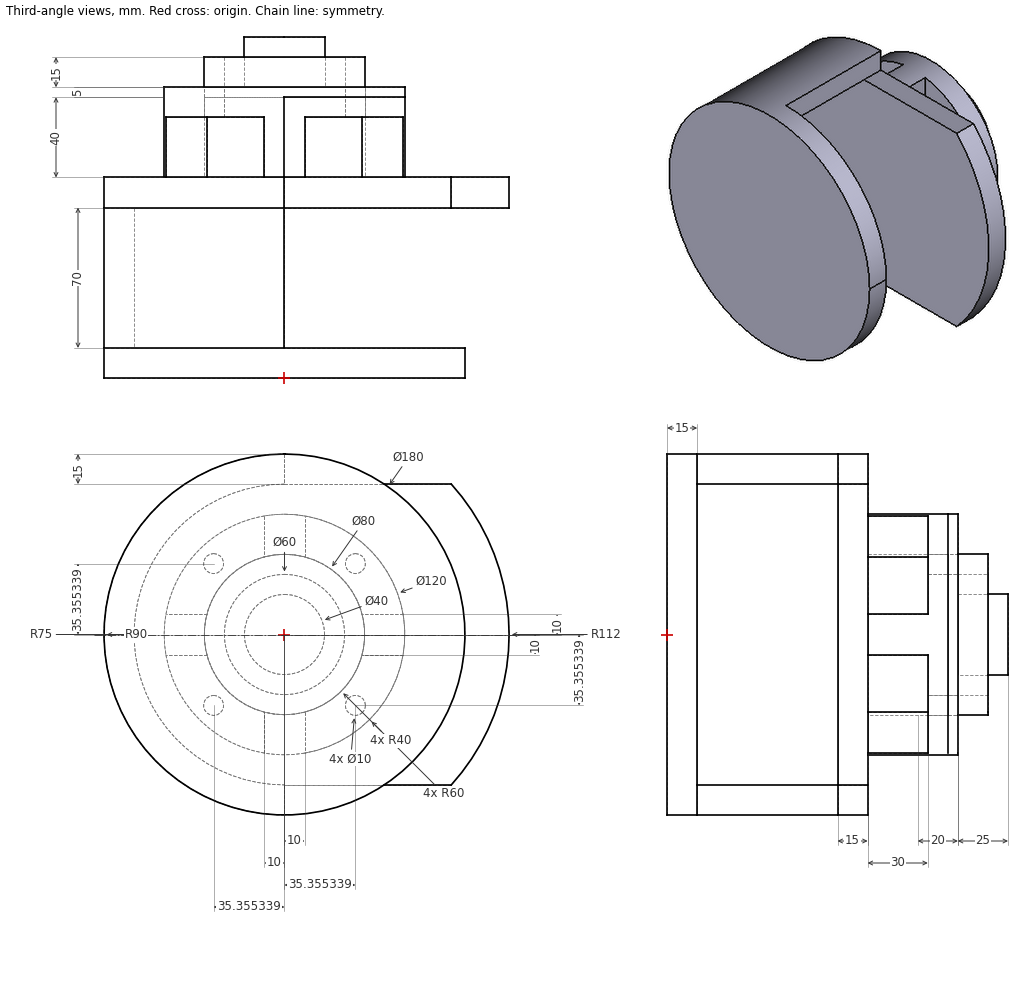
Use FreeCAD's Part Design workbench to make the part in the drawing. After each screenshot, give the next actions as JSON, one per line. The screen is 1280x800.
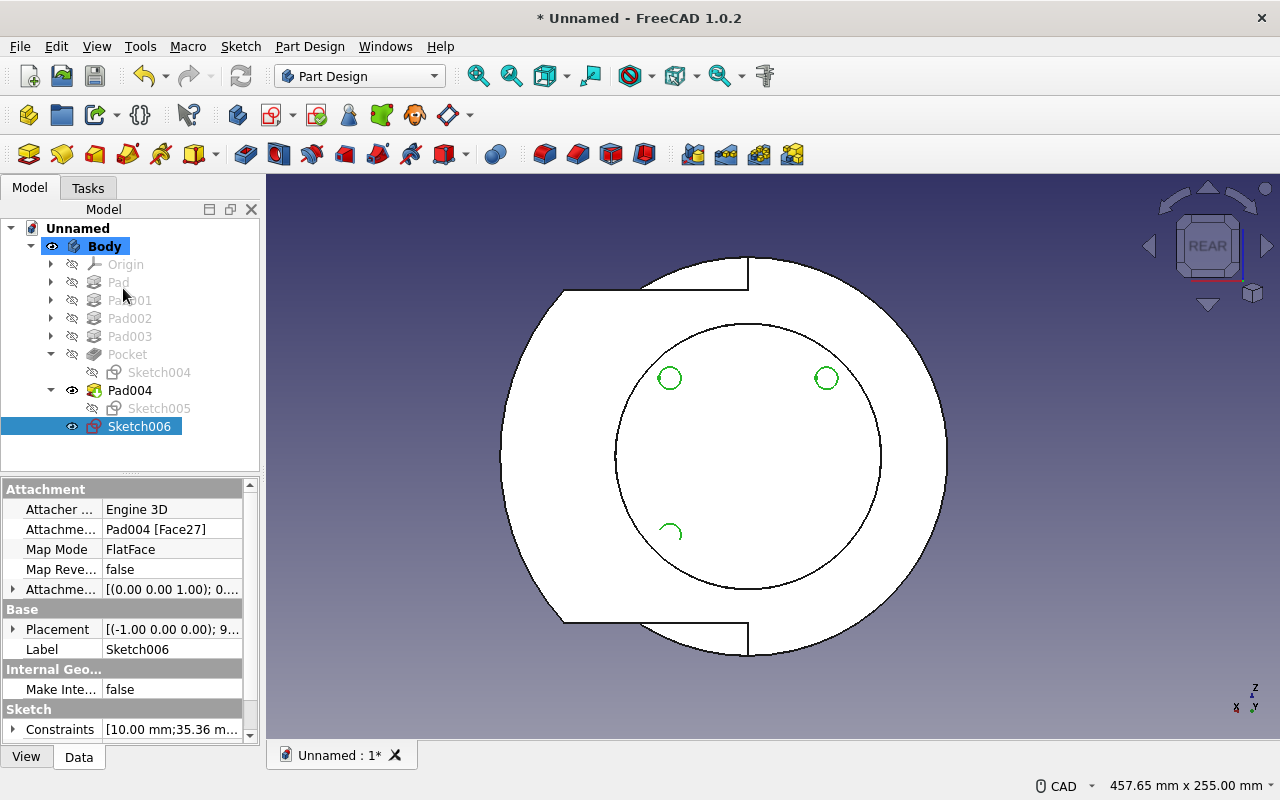
{"action": "left_click", "coordinate": [246, 154]}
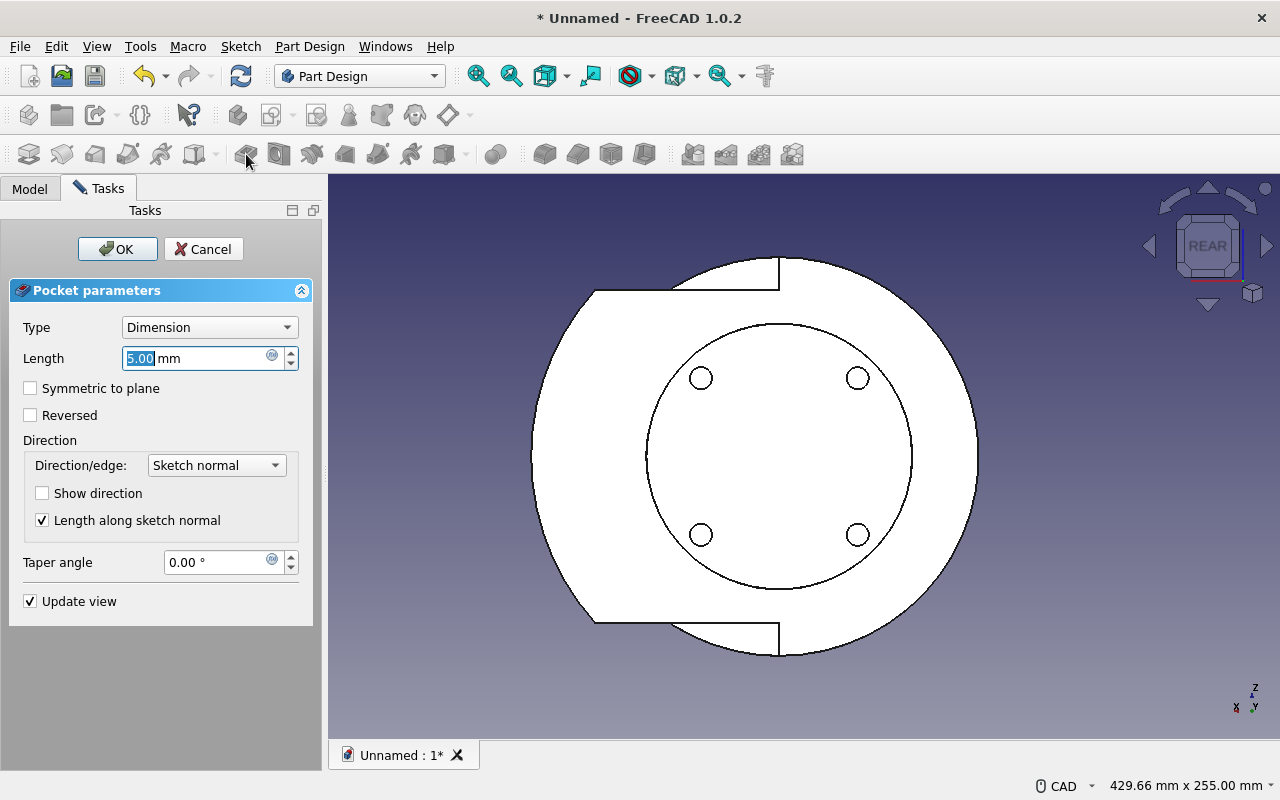
{"action": "type", "text": "20"}
{"action": "key", "text": "Tab"}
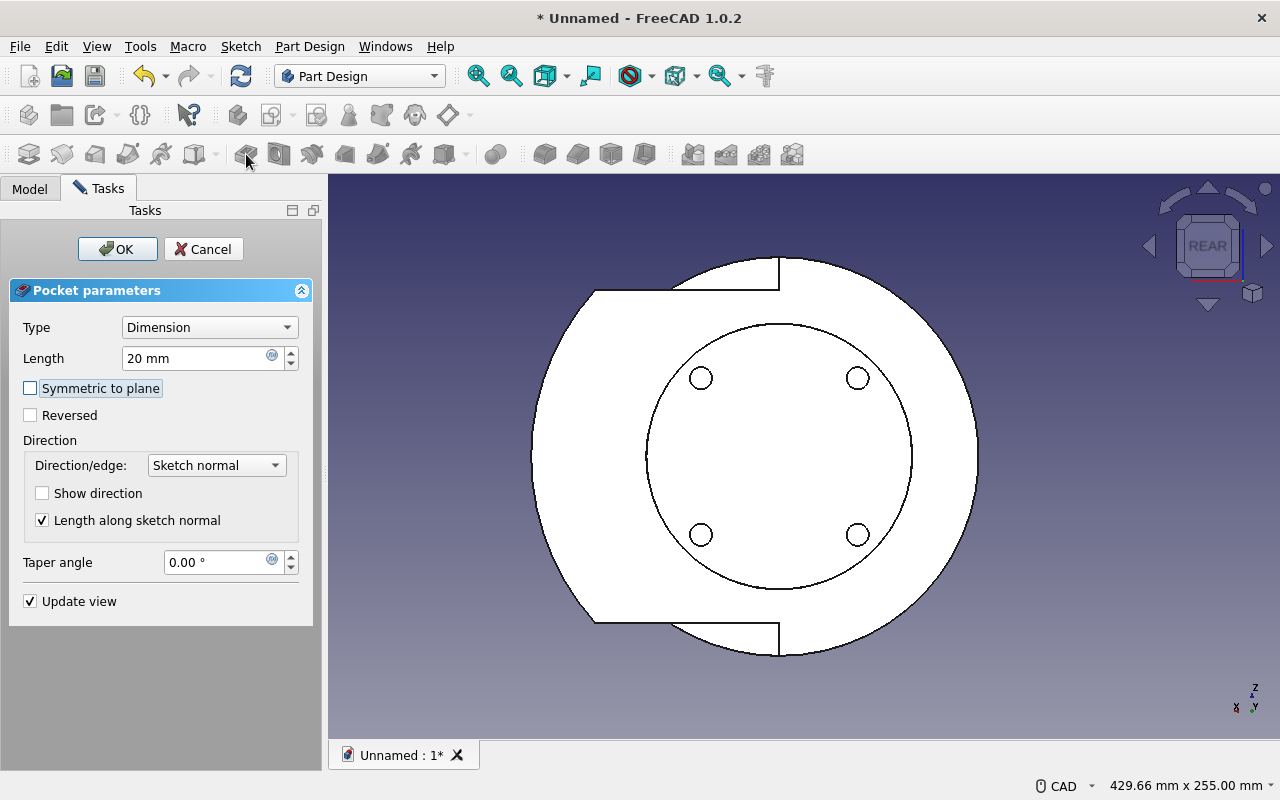
{"action": "left_click", "coordinate": [118, 249]}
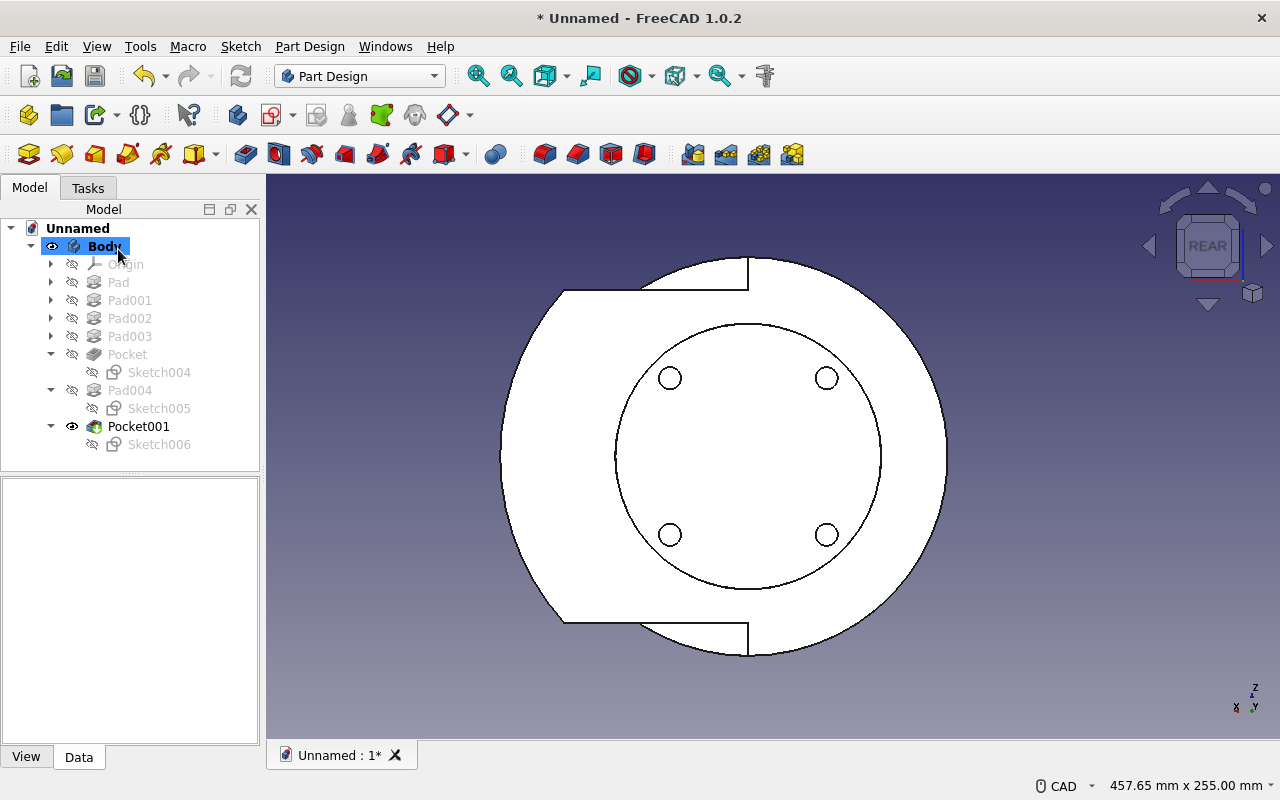
{"action": "left_click", "coordinate": [748, 455]}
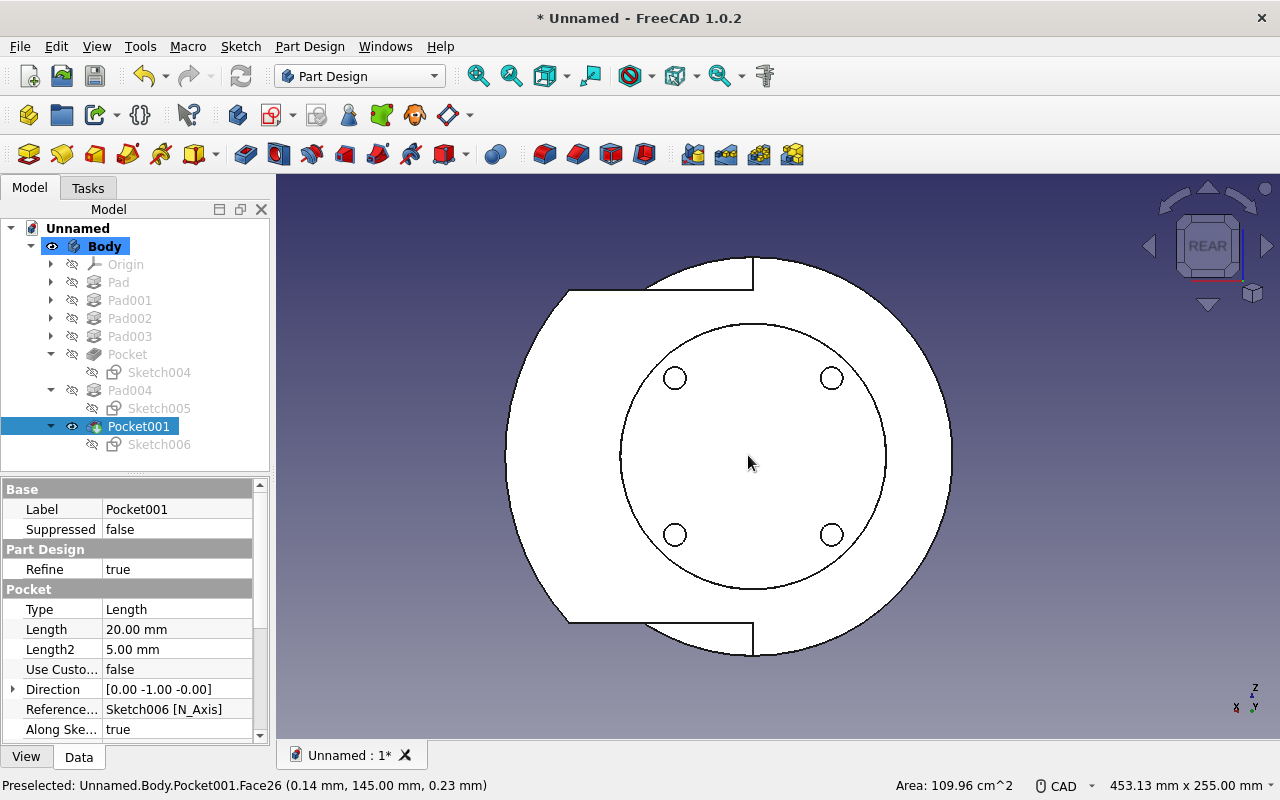
{"action": "left_click", "coordinate": [270, 116]}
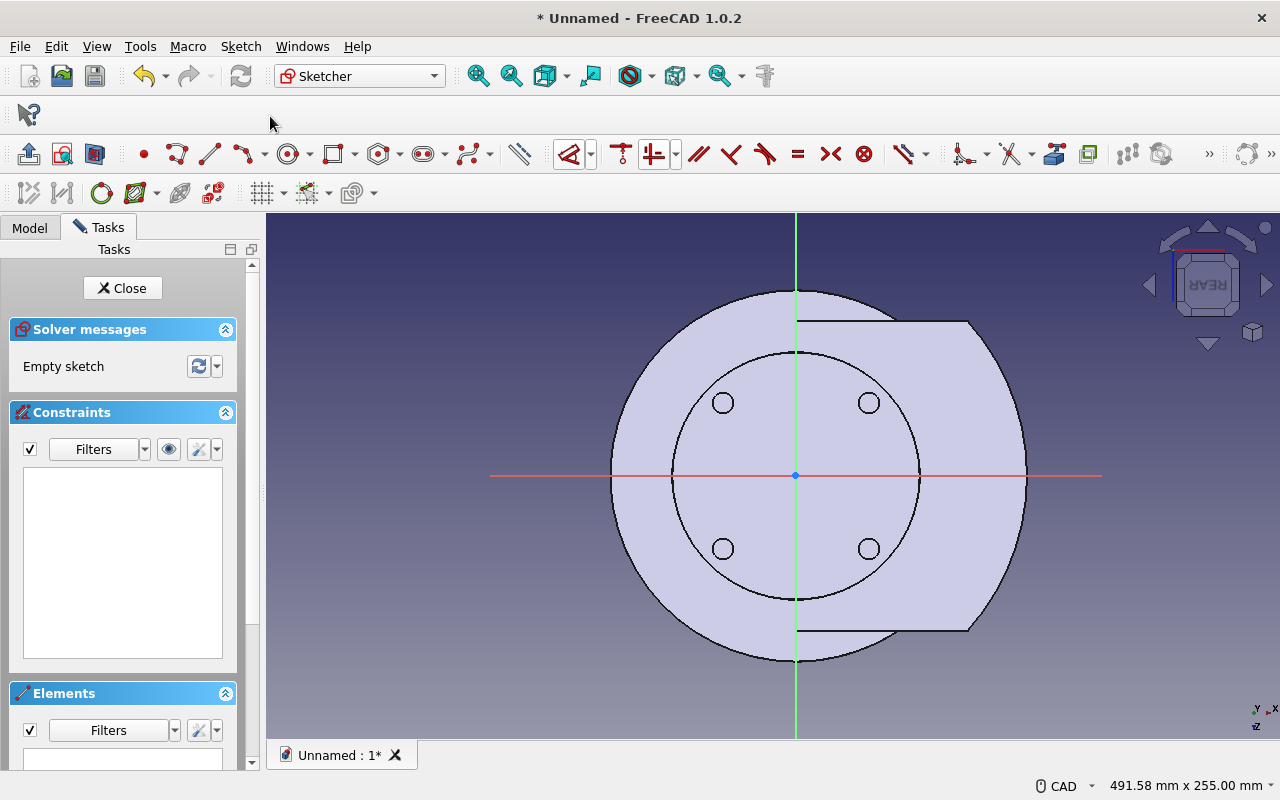
{"action": "scroll", "coordinate": [907, 476], "scroll_direction": "up", "scroll_amount": 3}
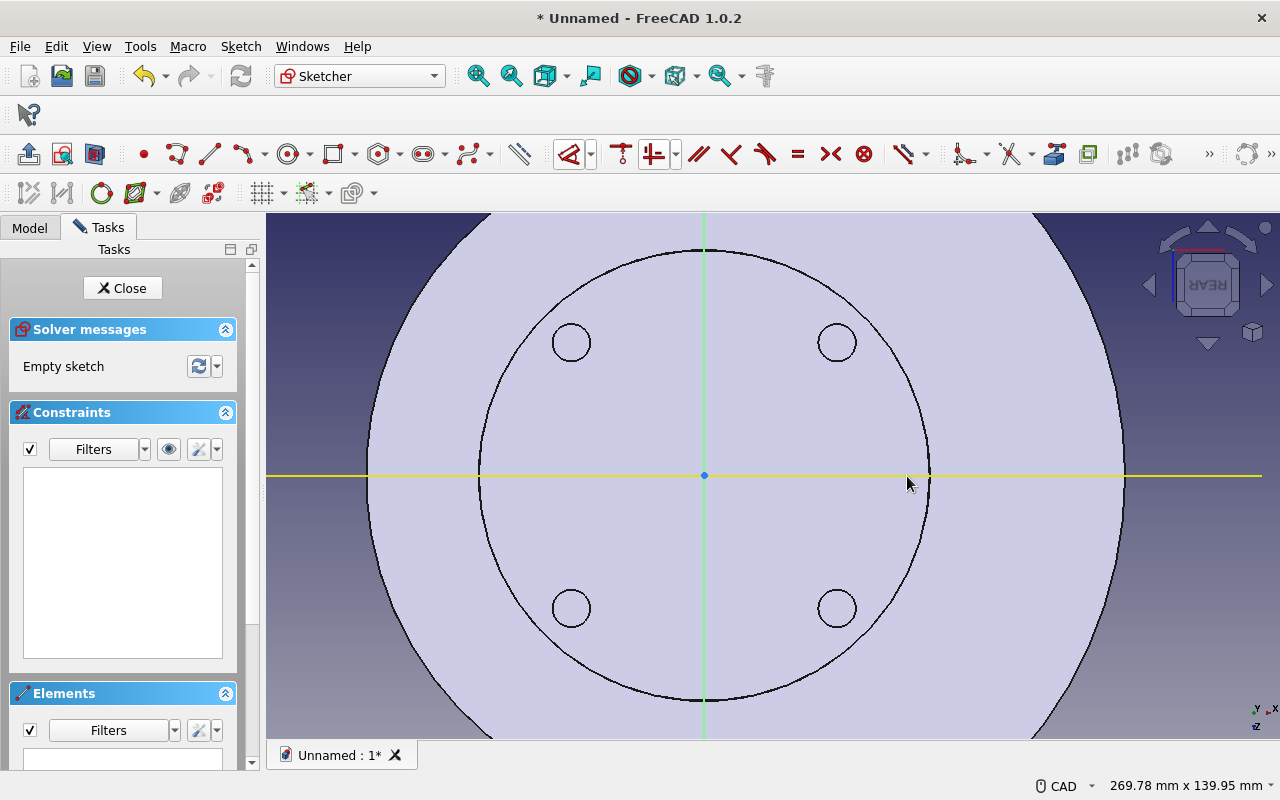
{"action": "key", "text": "g c"}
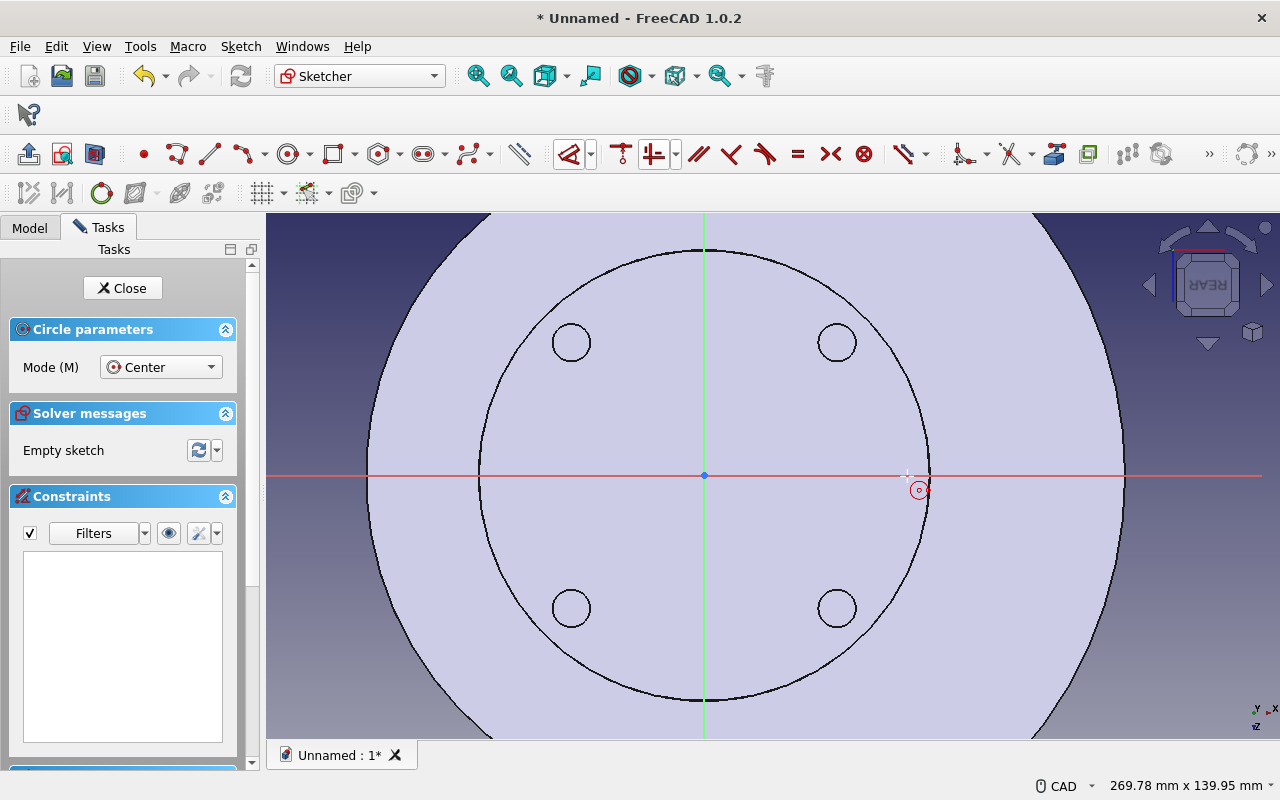
{"action": "left_click", "coordinate": [704, 476]}
{"action": "left_click", "coordinate": [811, 369]}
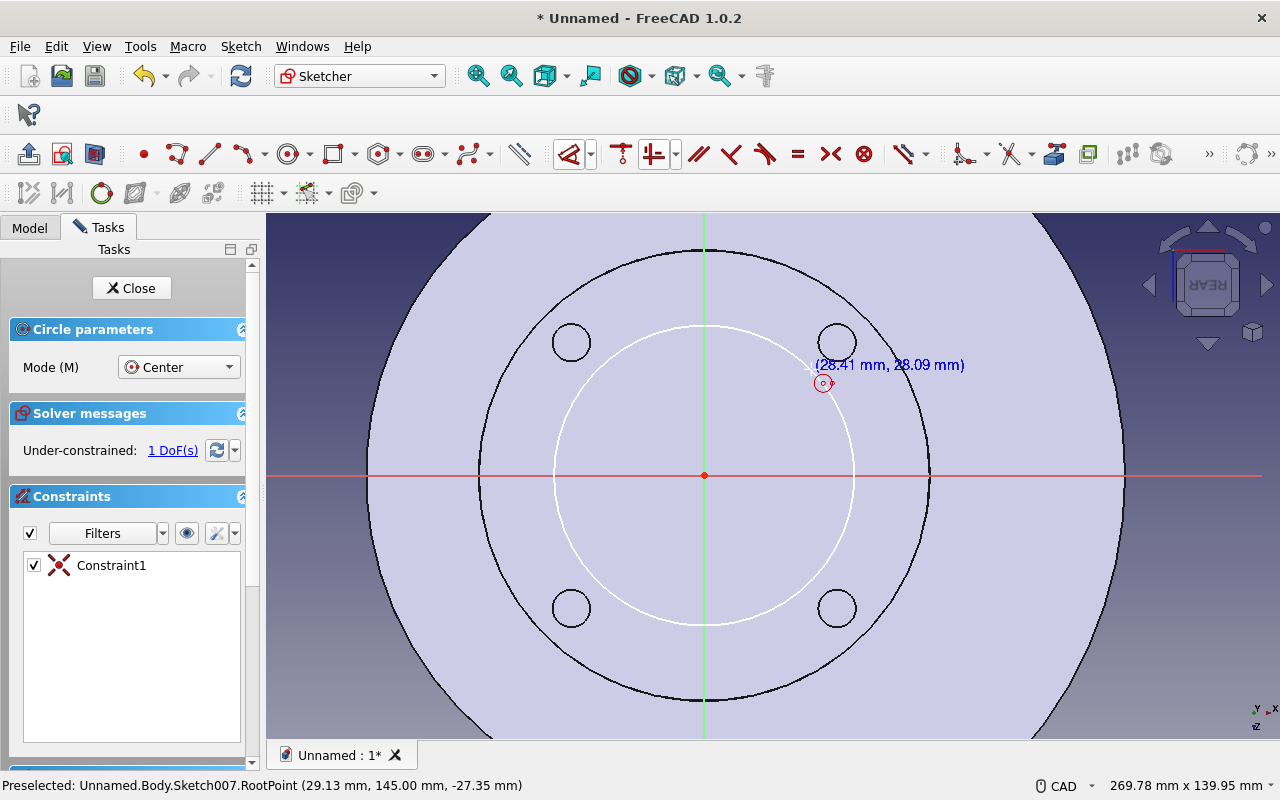
{"action": "left_click", "coordinate": [704, 476]}
{"action": "left_click", "coordinate": [784, 396]}
{"action": "key", "text": "Escape"}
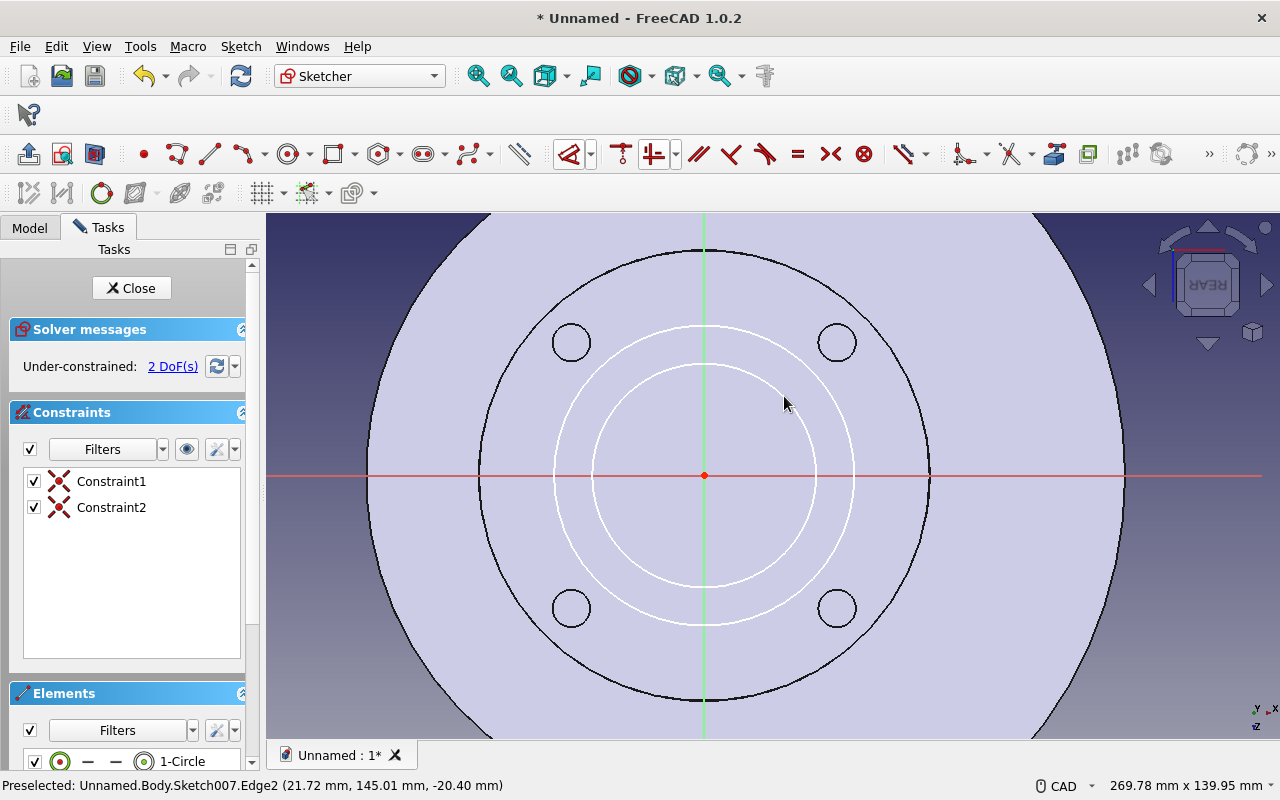
{"action": "left_click", "coordinate": [810, 369]}